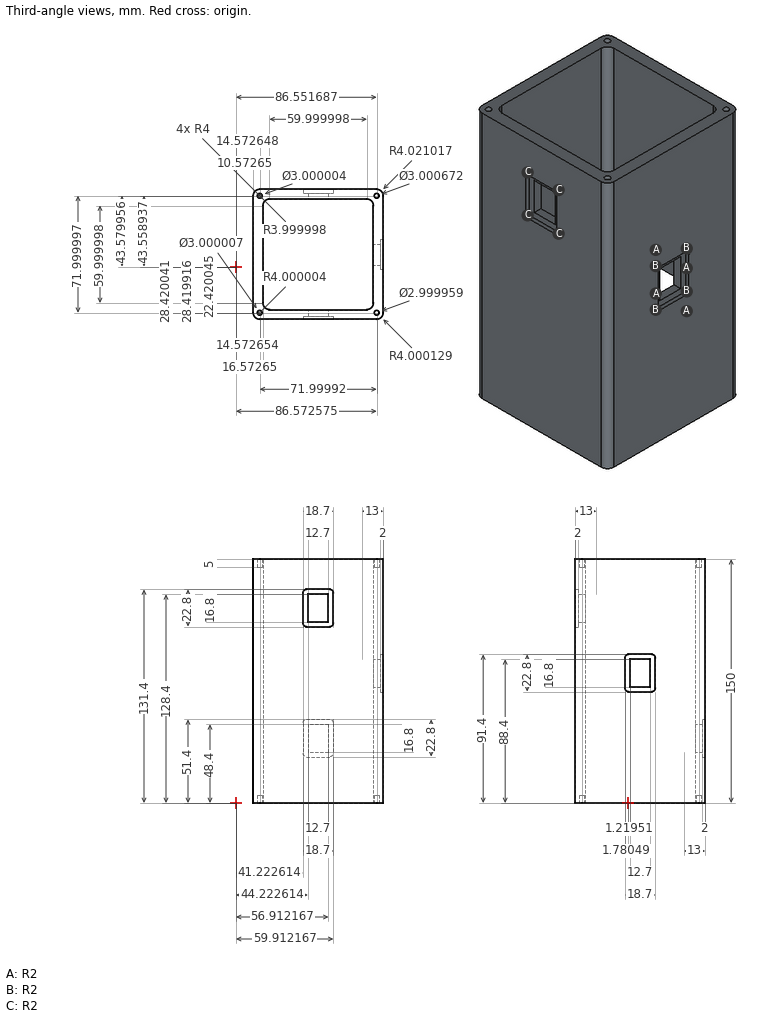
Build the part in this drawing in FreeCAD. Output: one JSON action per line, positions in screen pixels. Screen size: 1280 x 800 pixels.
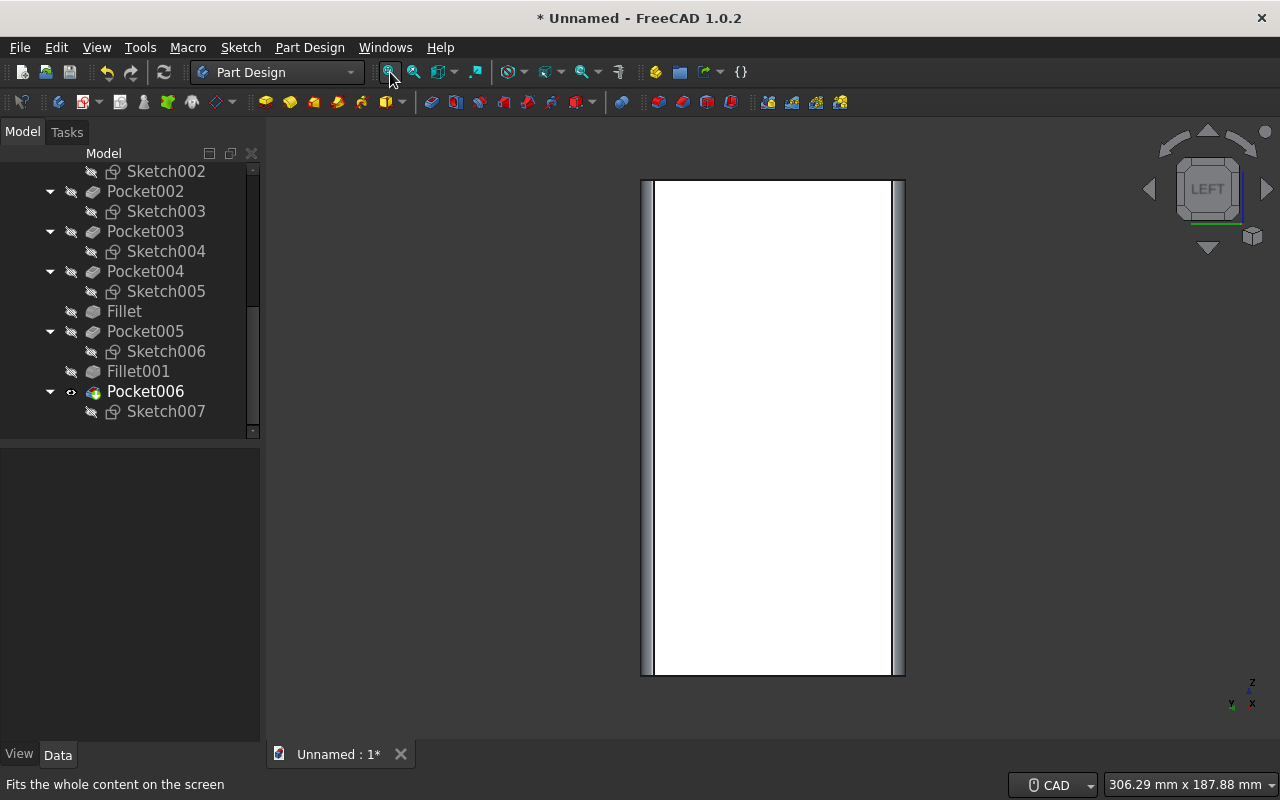
{"action": "scroll", "coordinate": [902, 316], "scroll_direction": "up", "scroll_amount": 9}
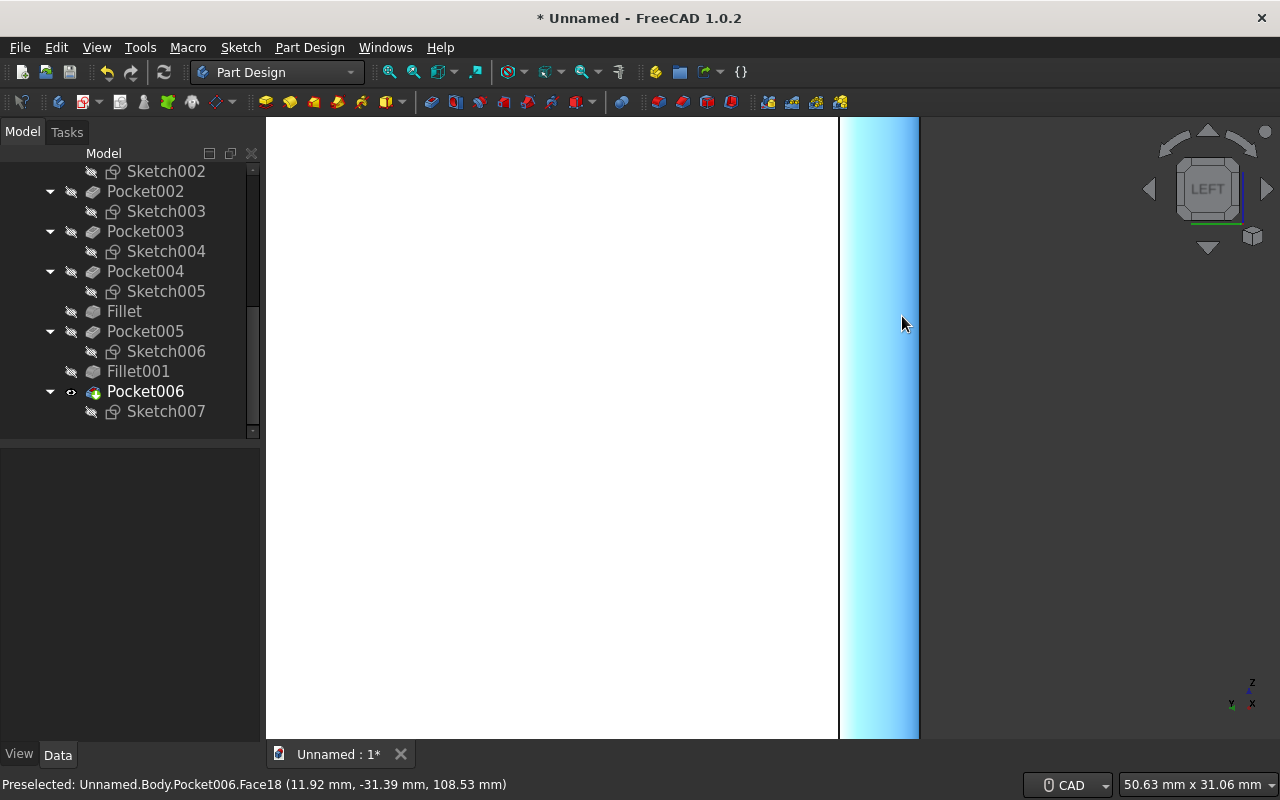
{"action": "left_click", "coordinate": [390, 72]}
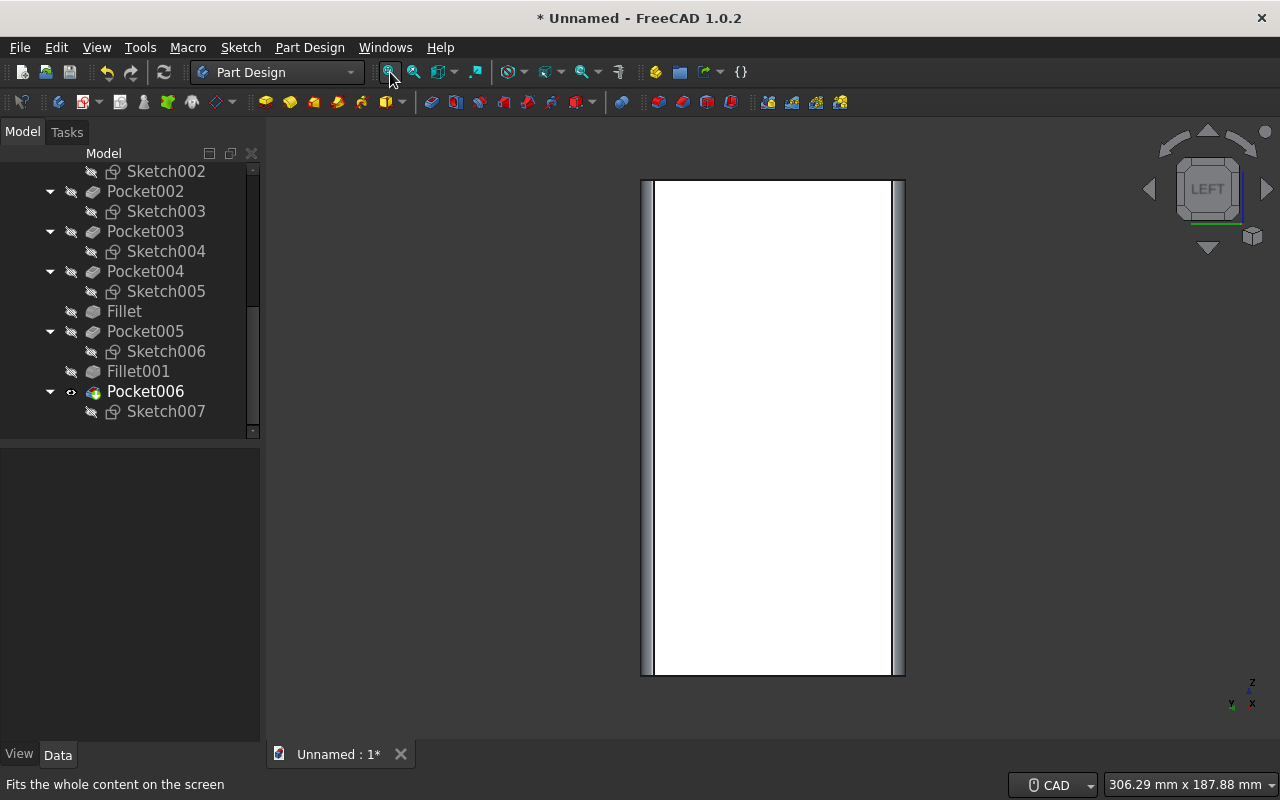
{"action": "key", "text": "v 3"}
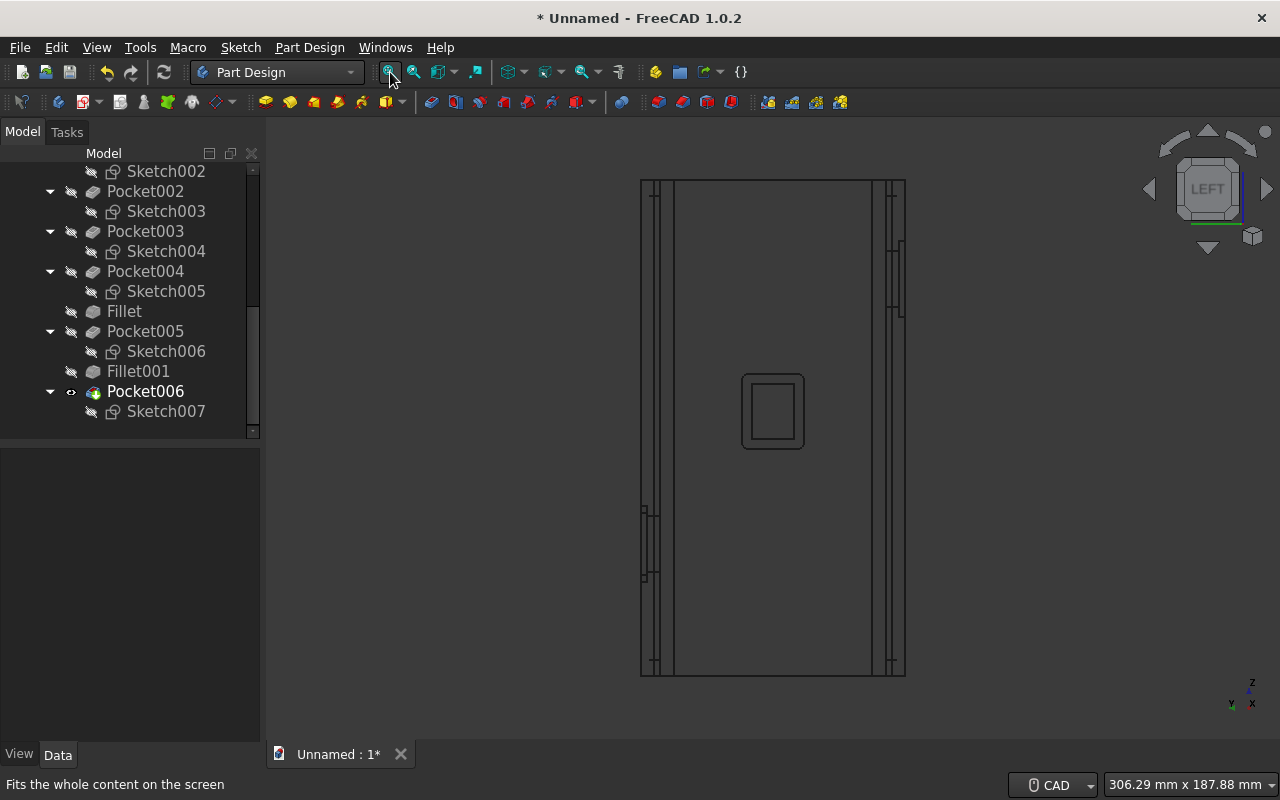
{"action": "key", "text": "0"}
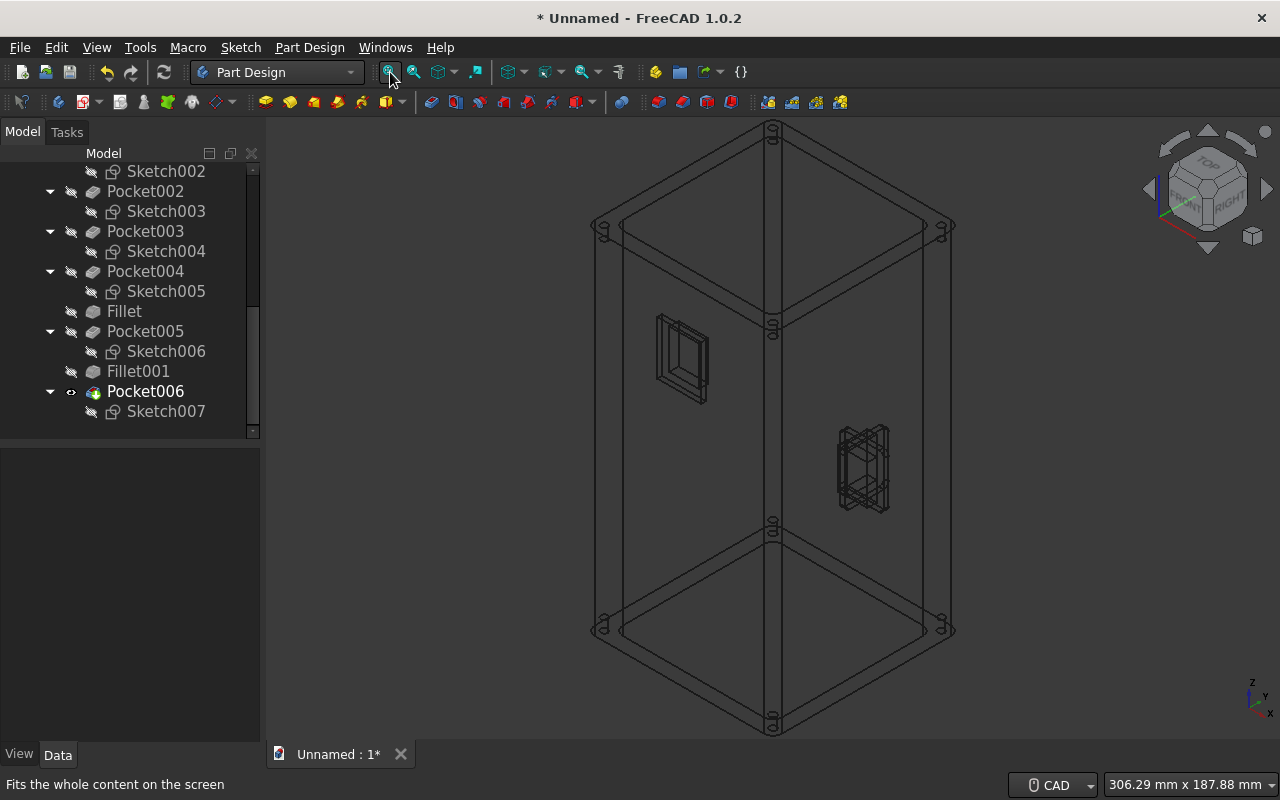
{"action": "key", "text": "v f"}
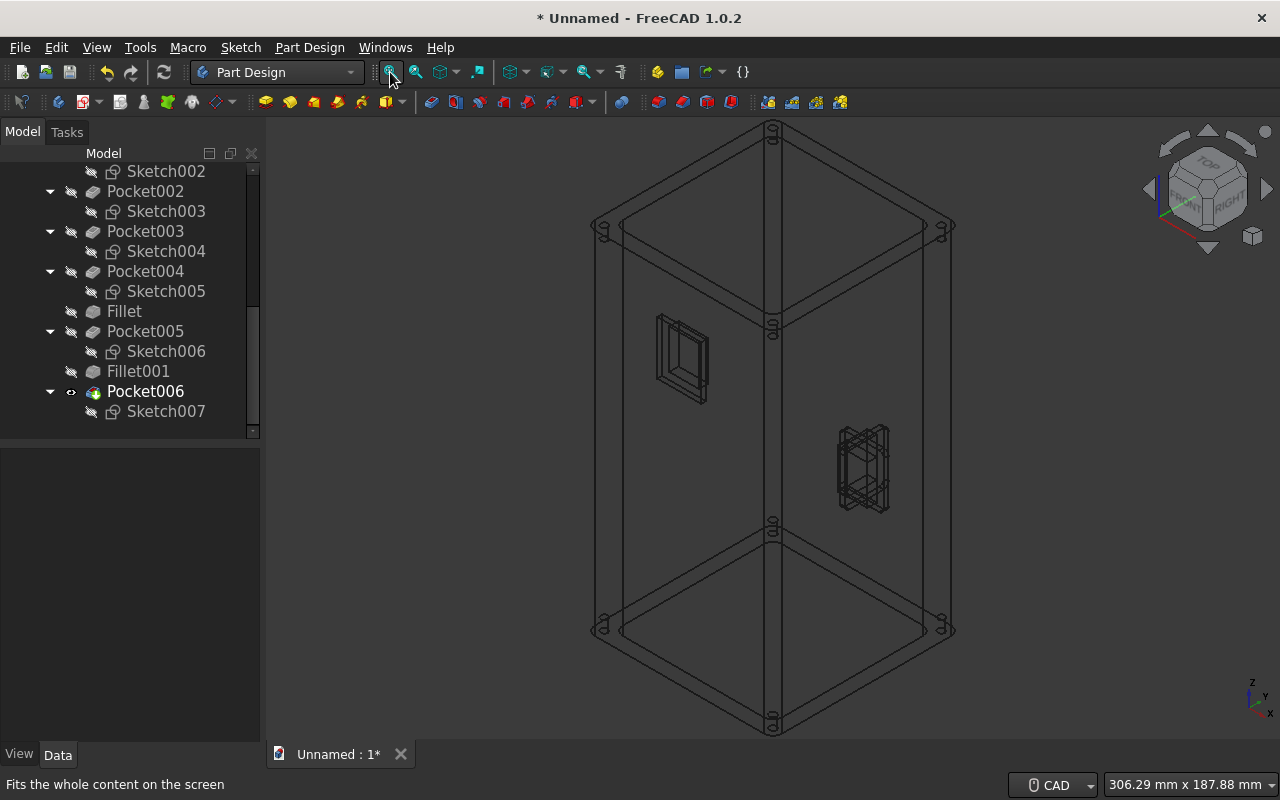
{"action": "scroll", "coordinate": [660, 376], "scroll_direction": "up", "scroll_amount": 9}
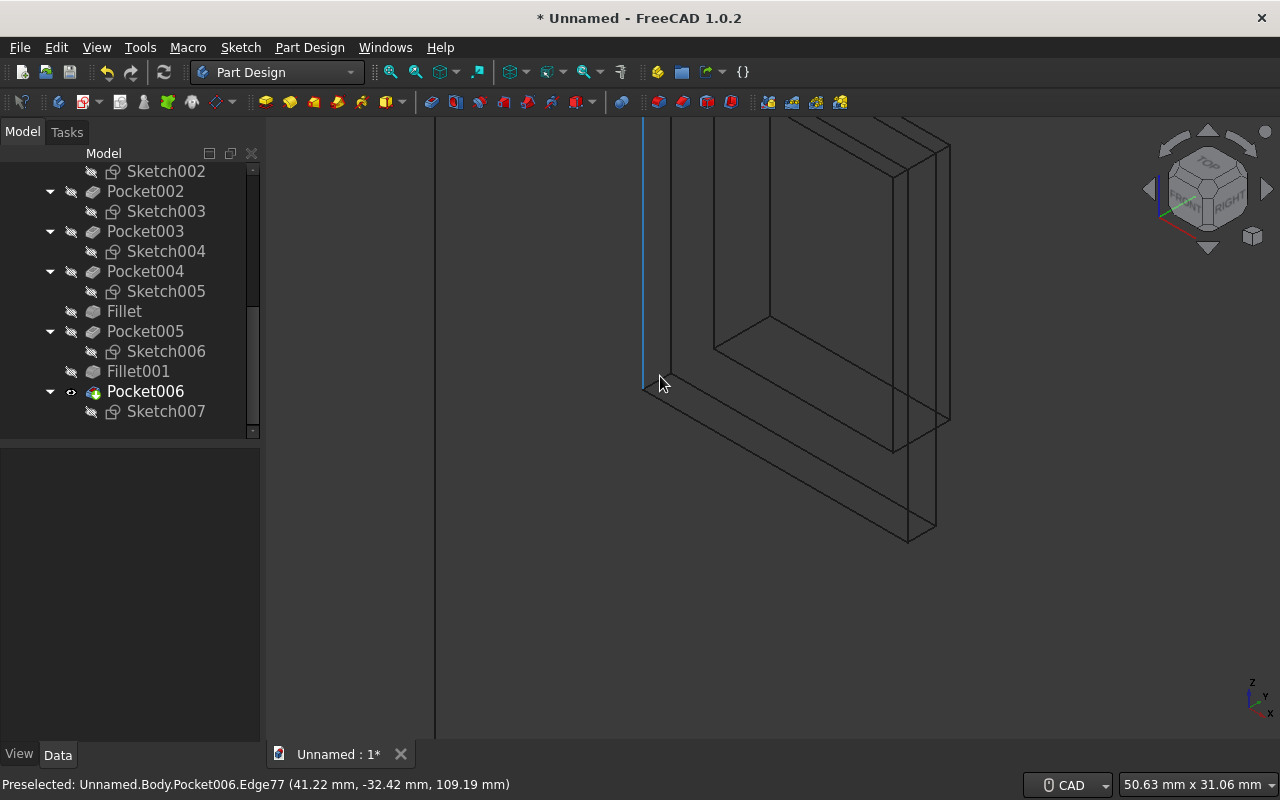
{"action": "left_click", "coordinate": [657, 380]}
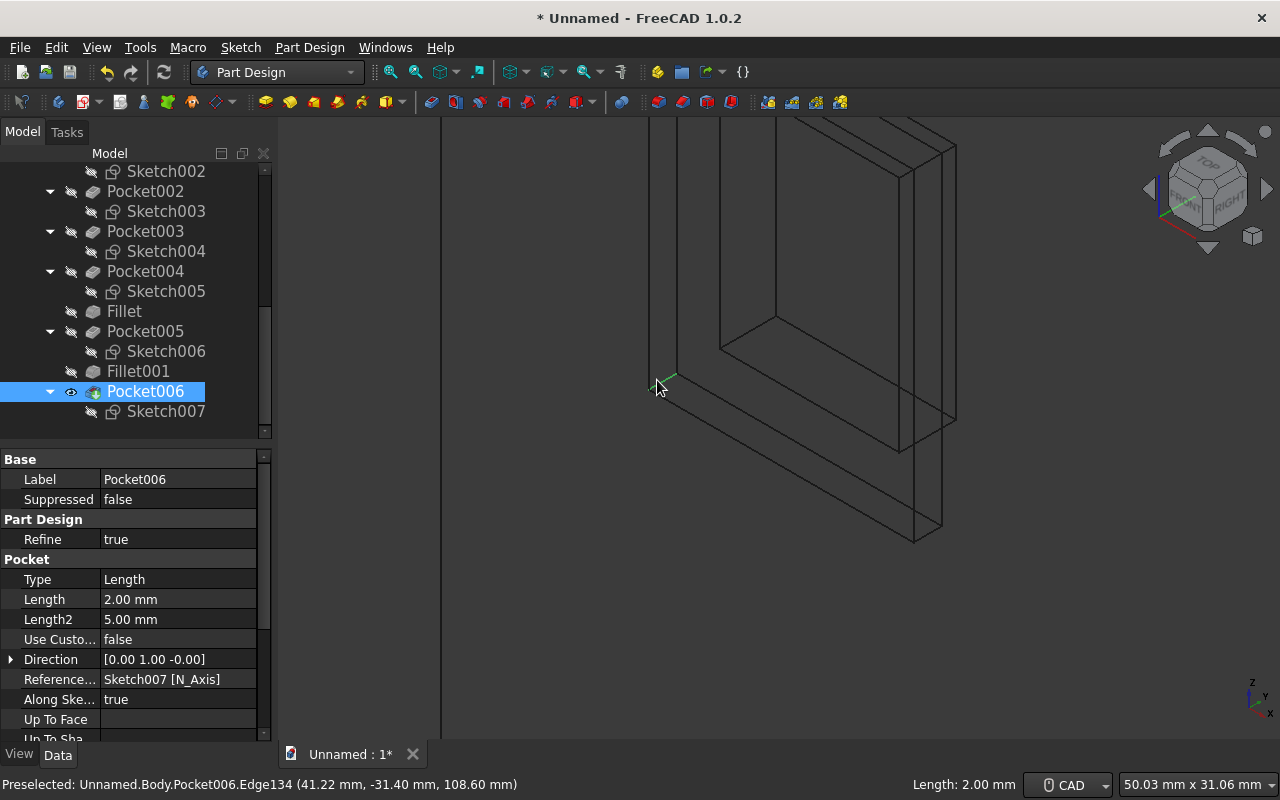
{"action": "left_click", "coordinate": [928, 161], "text": "ctrl"}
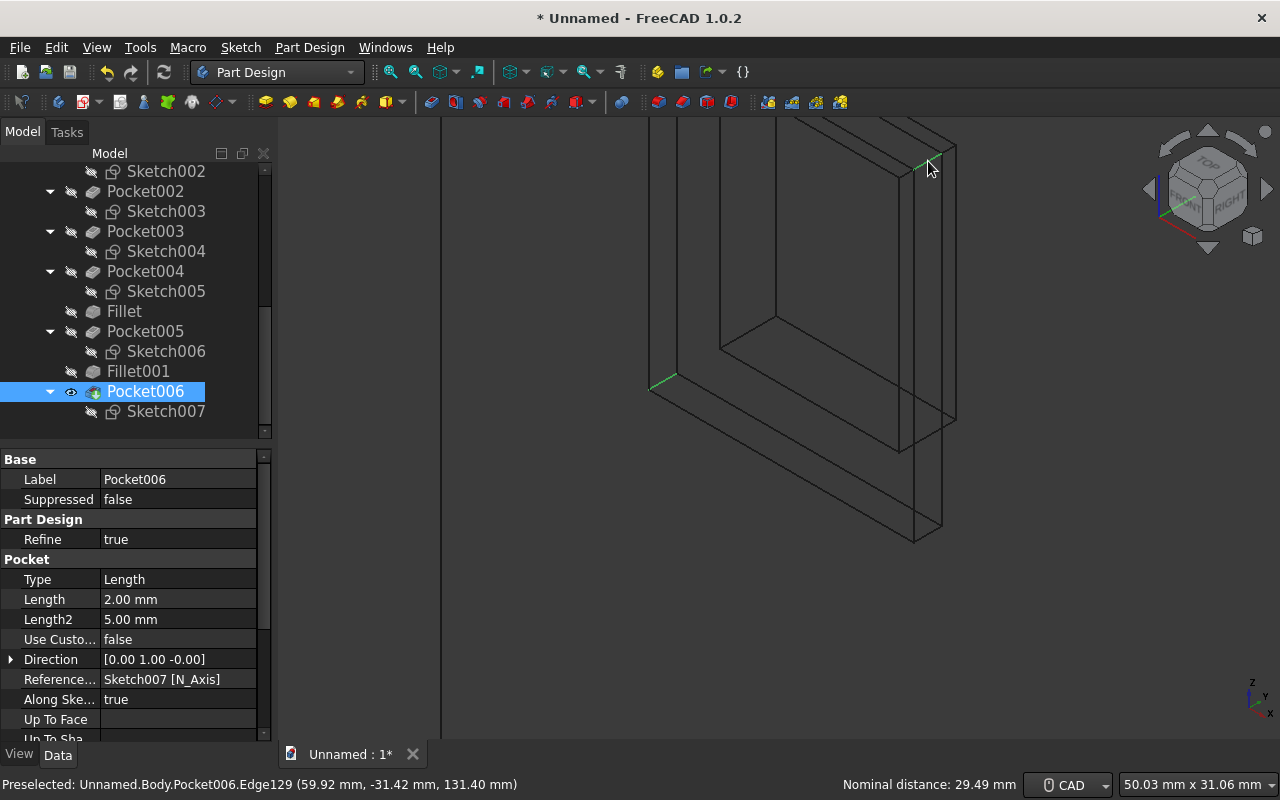
{"action": "left_click", "coordinate": [928, 533], "text": "ctrl"}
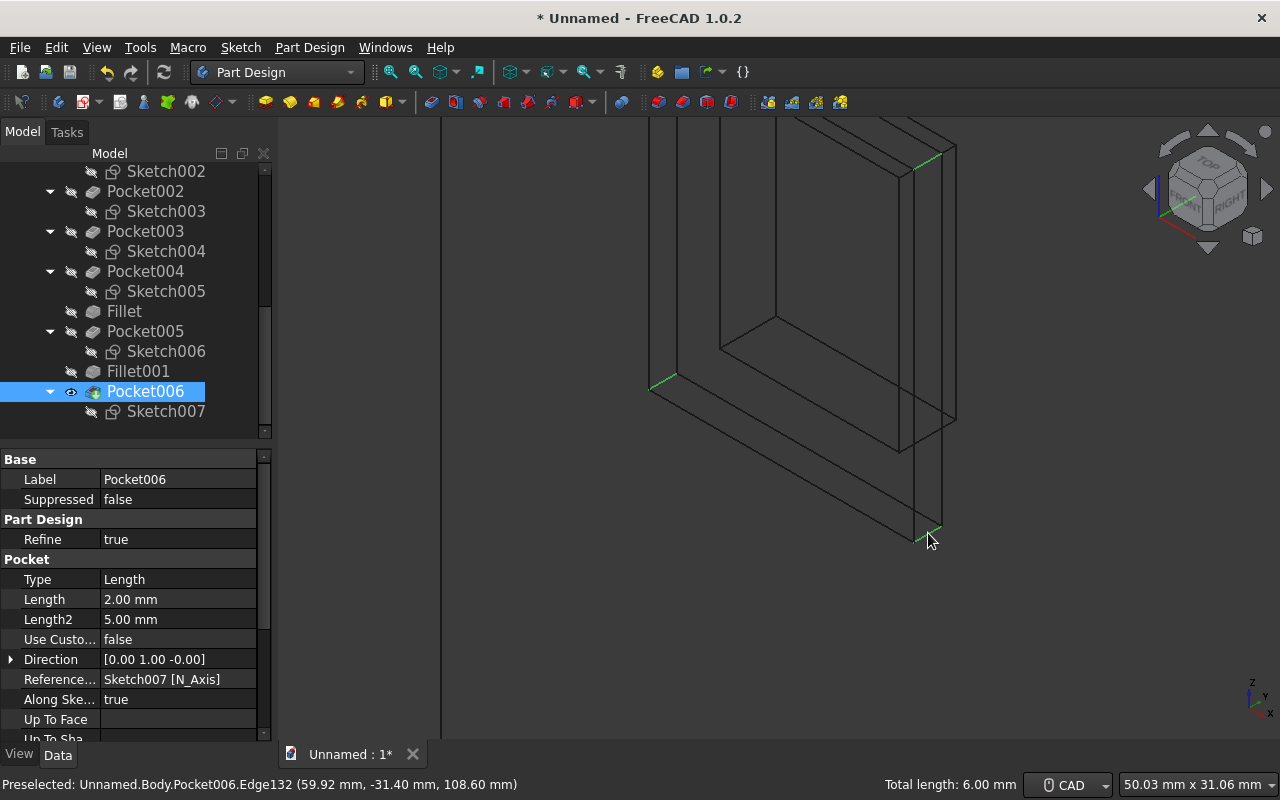
{"action": "key", "text": "v f"}